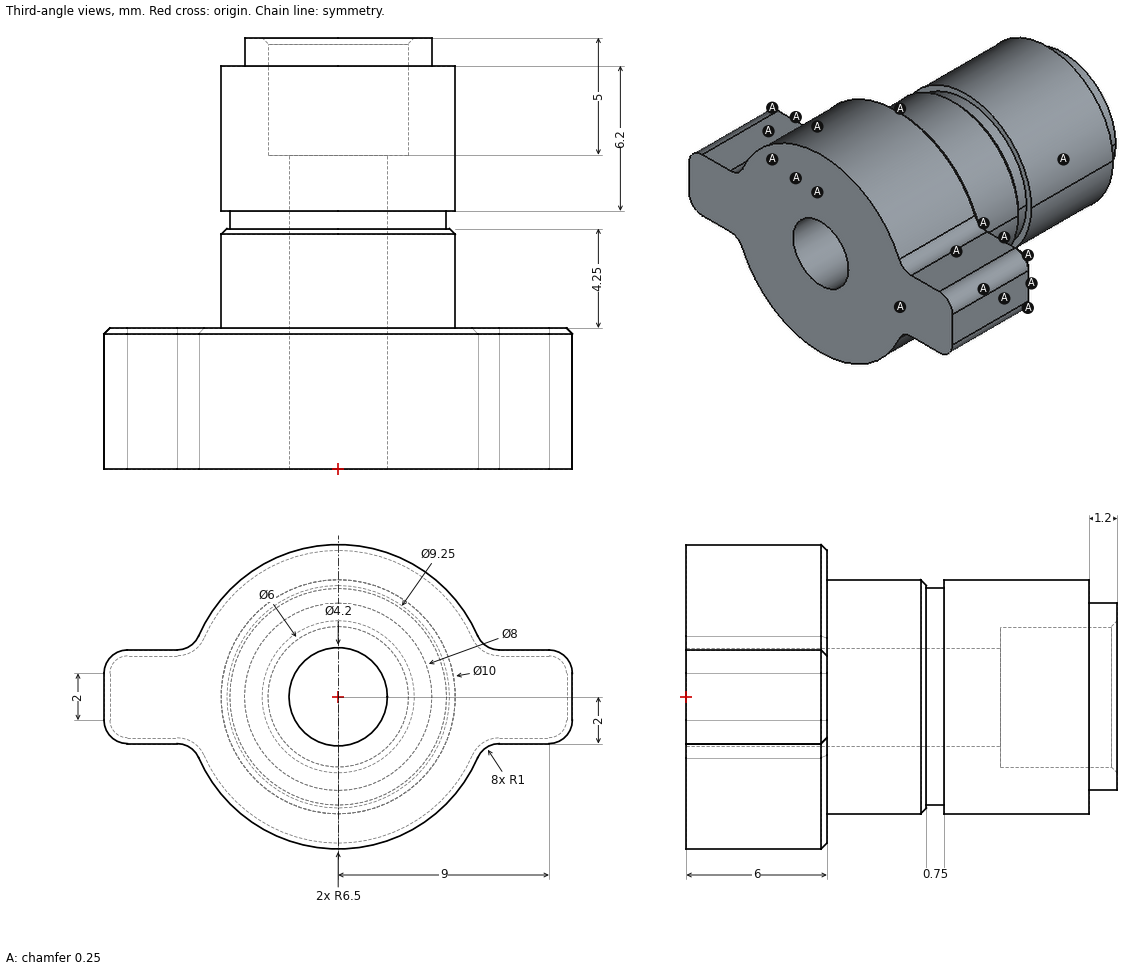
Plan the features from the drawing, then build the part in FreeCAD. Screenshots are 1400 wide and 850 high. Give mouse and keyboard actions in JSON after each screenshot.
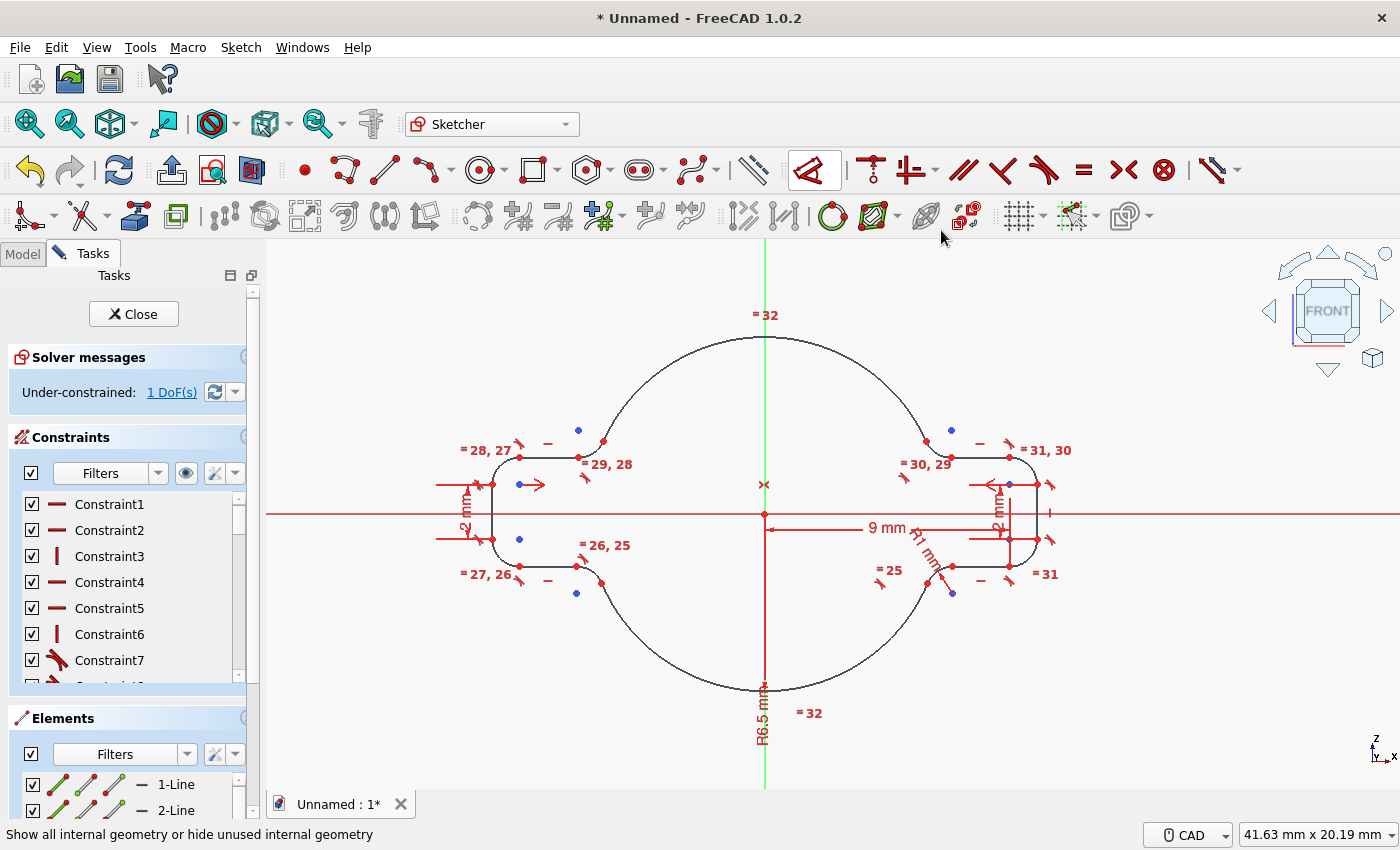
{"action": "left_click", "coordinate": [1010, 567]}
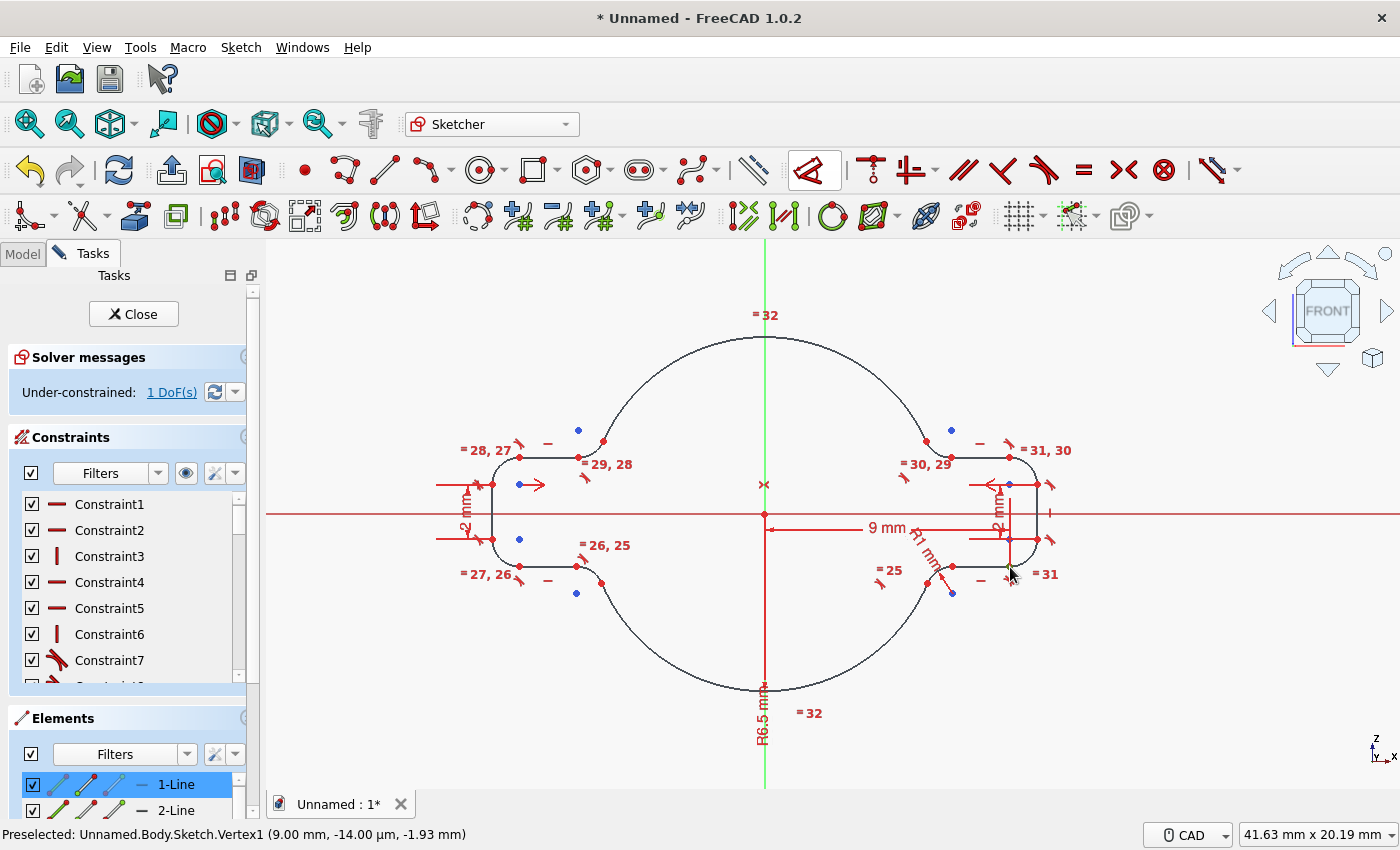
{"action": "key", "text": "i"}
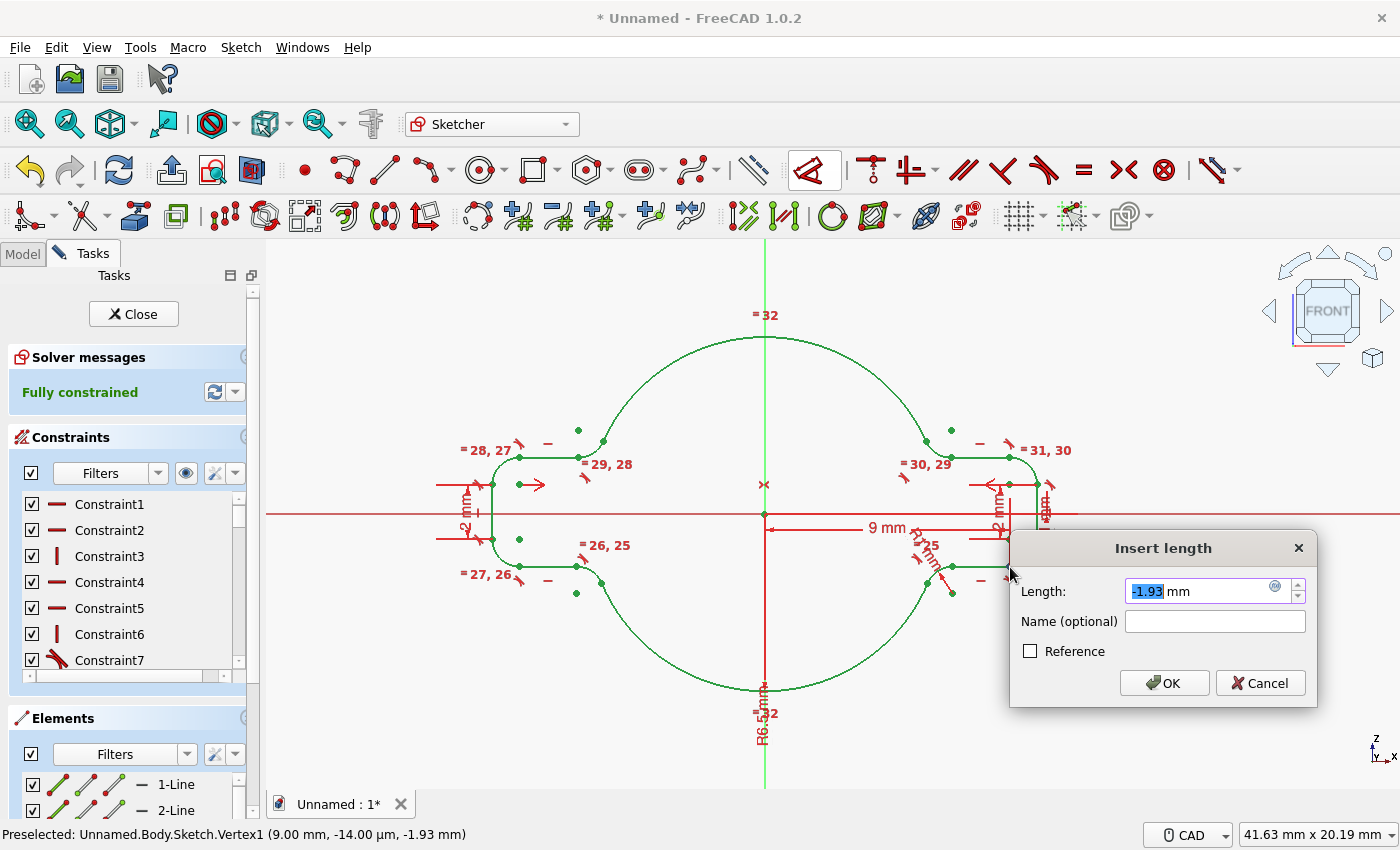
{"action": "type", "text": "-2"}
{"action": "key", "text": "Return"}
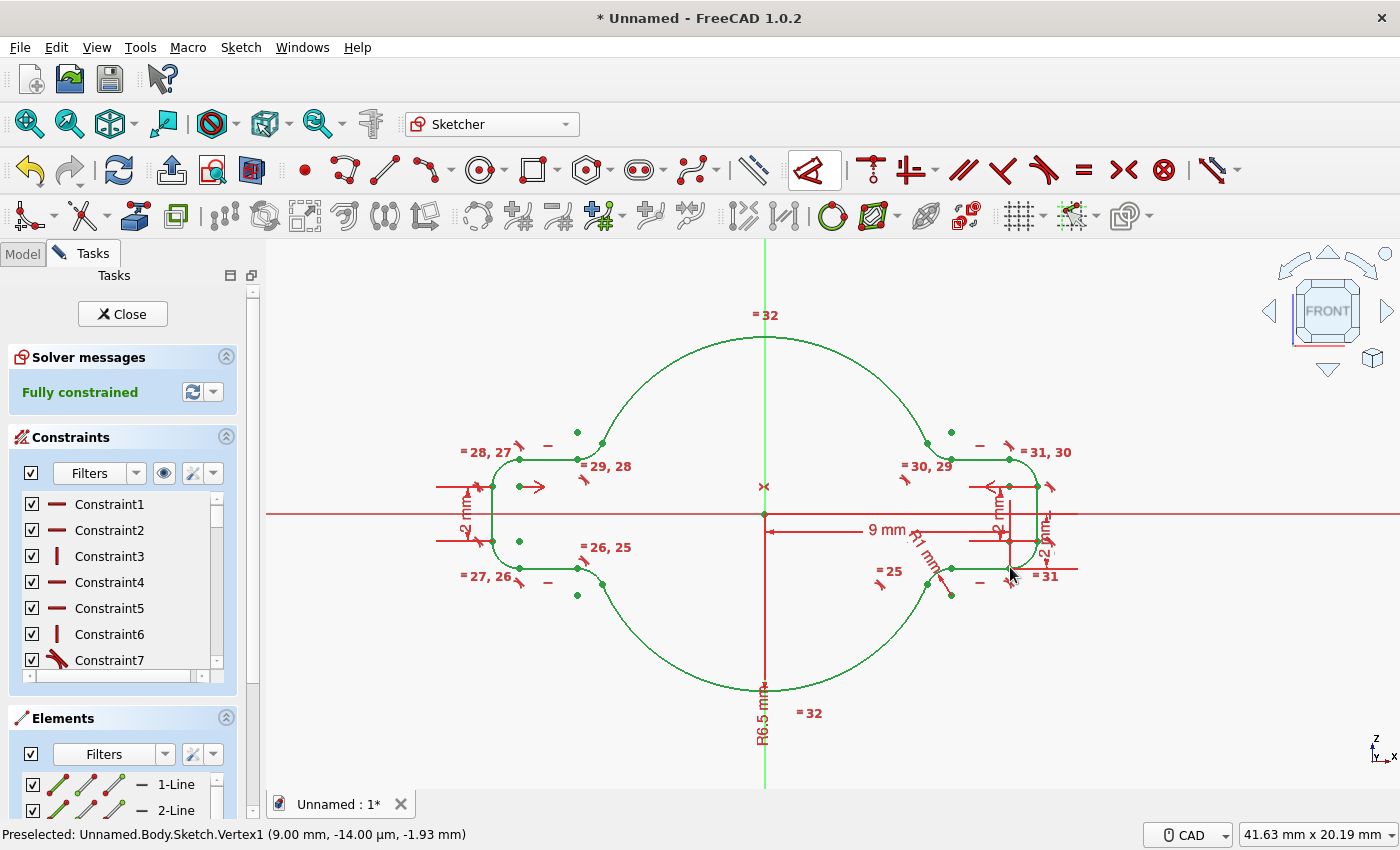
{"action": "left_click", "coordinate": [123, 314]}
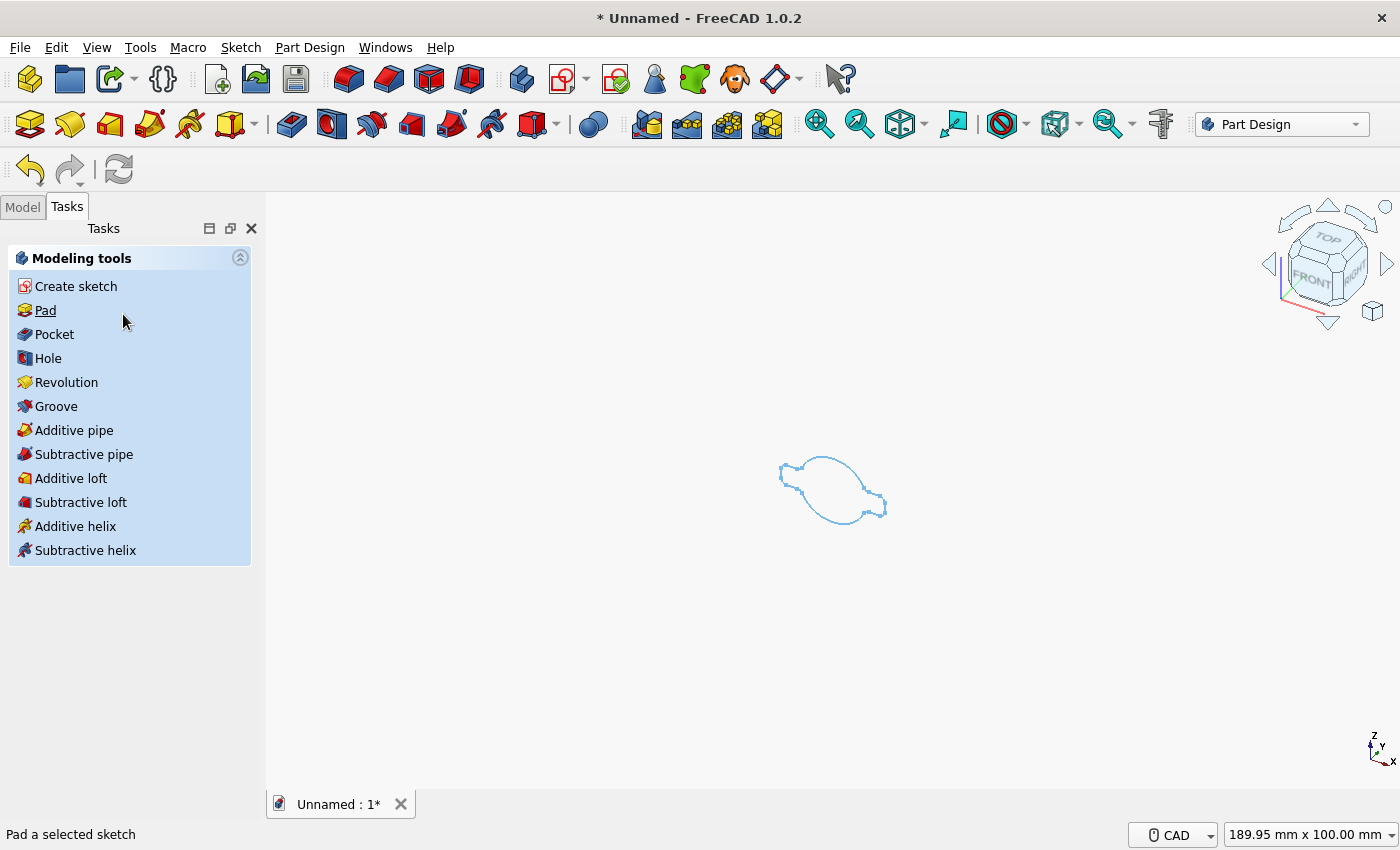
{"action": "left_click", "coordinate": [30, 124]}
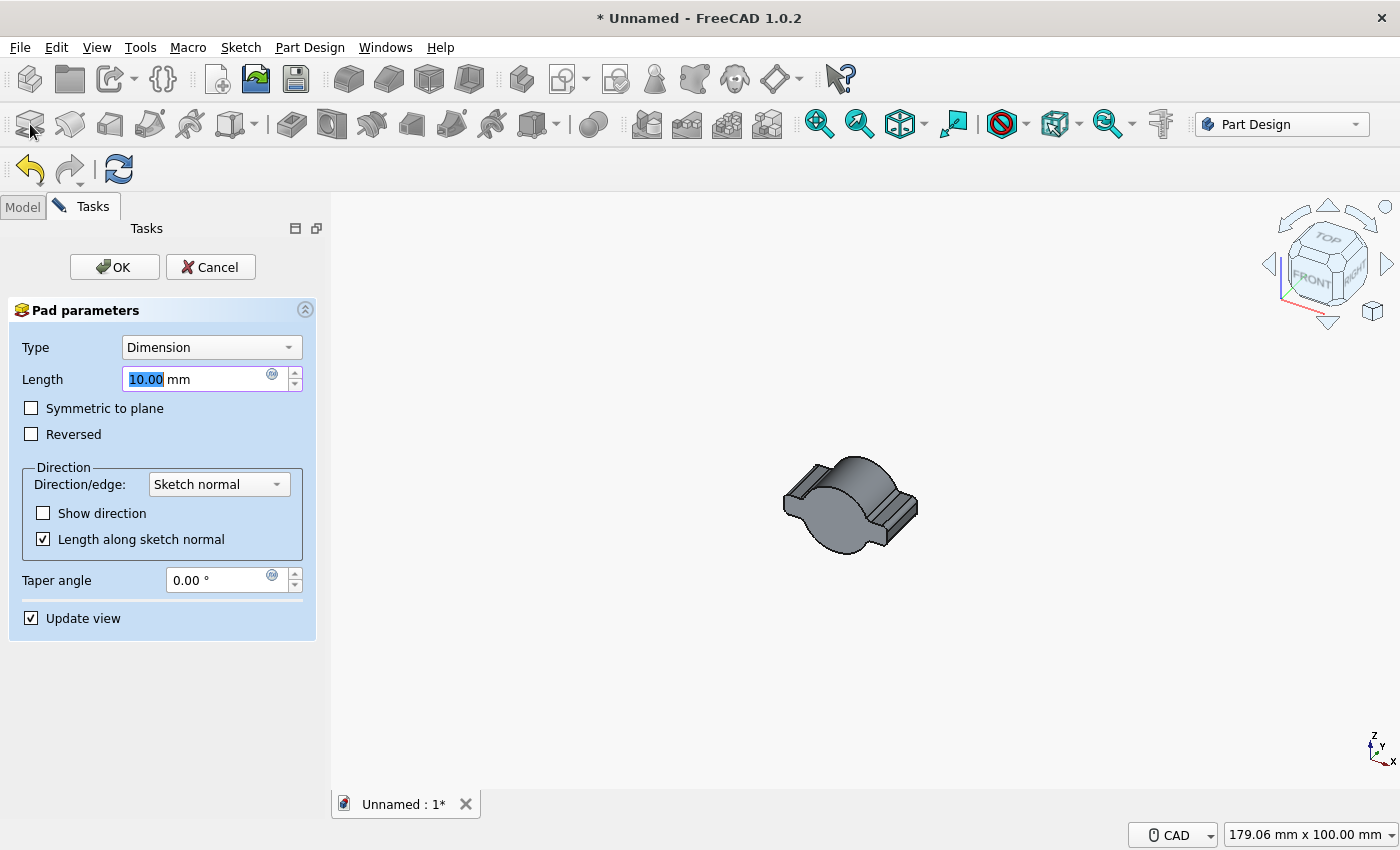
{"action": "type", "text": "6"}
{"action": "key", "text": "Tab"}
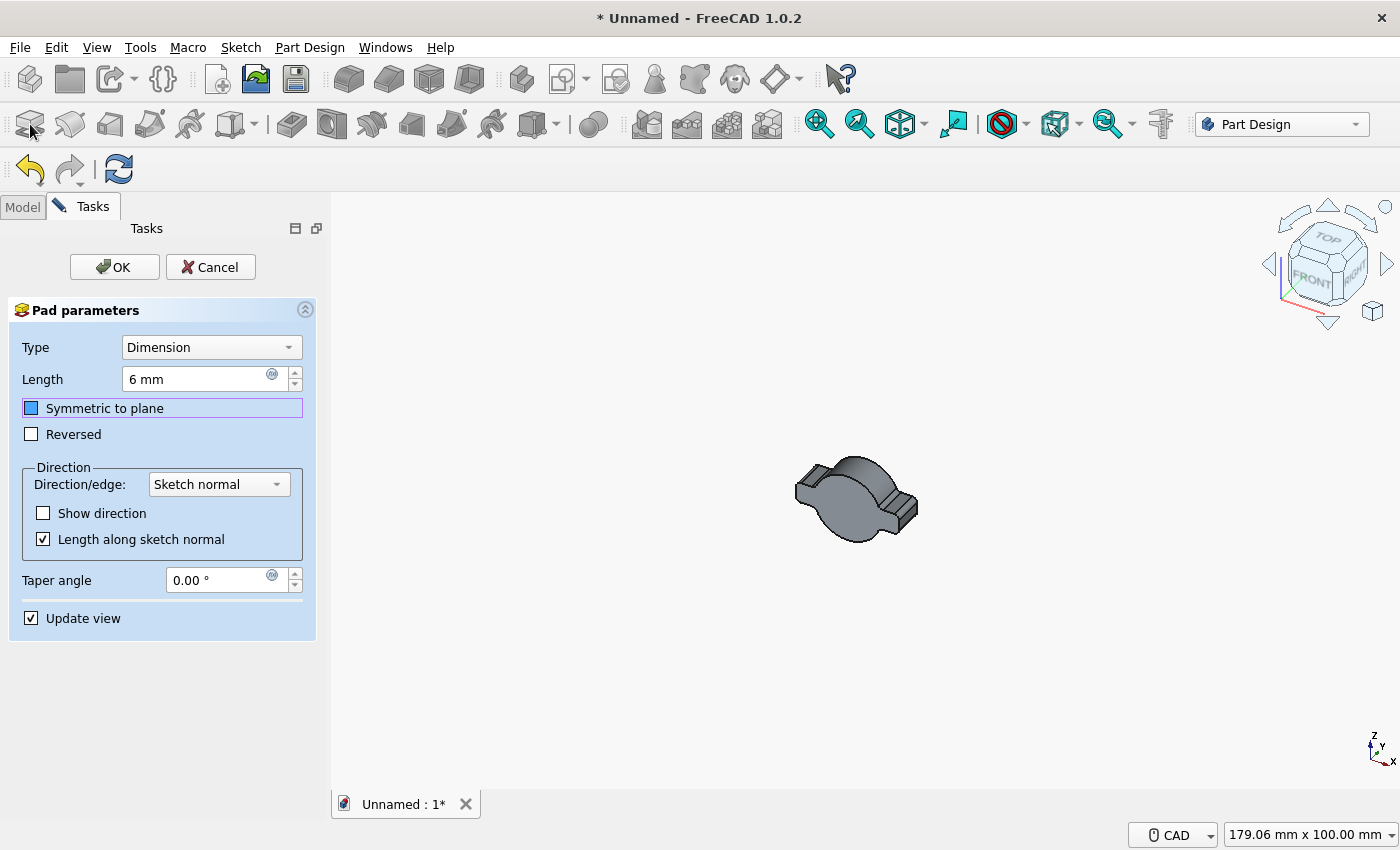
{"action": "left_click", "coordinate": [30, 434]}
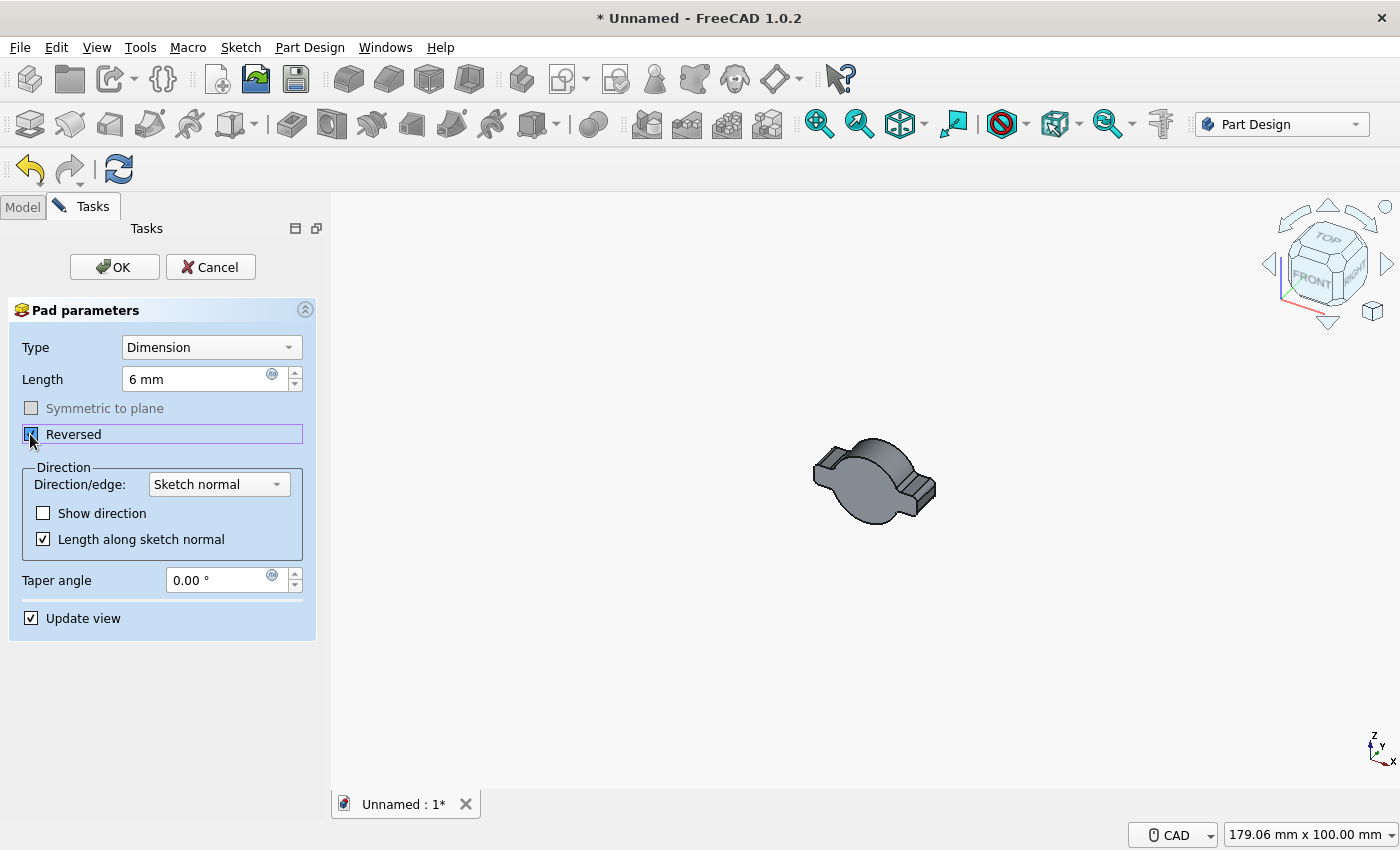
{"action": "left_click", "coordinate": [115, 267]}